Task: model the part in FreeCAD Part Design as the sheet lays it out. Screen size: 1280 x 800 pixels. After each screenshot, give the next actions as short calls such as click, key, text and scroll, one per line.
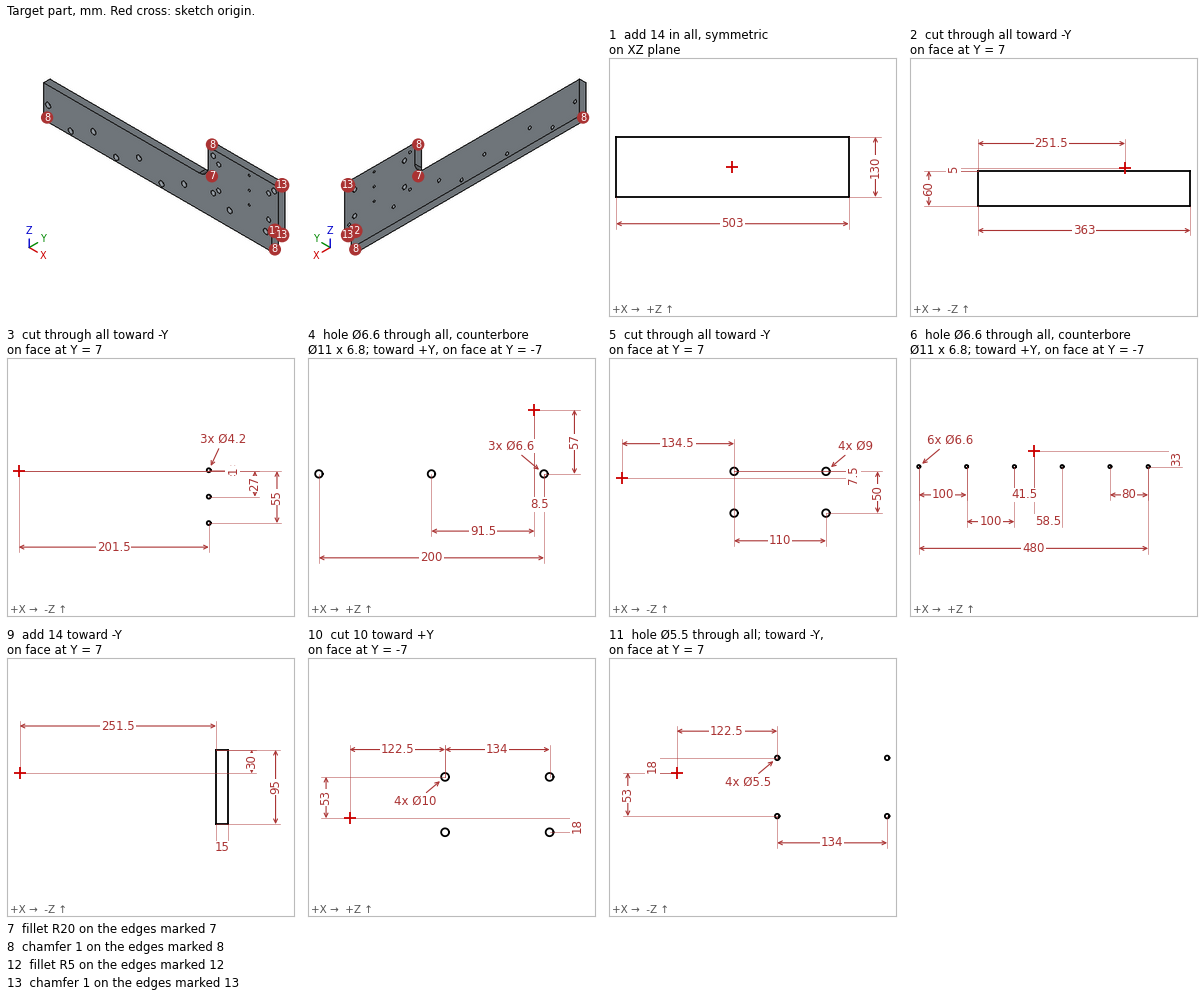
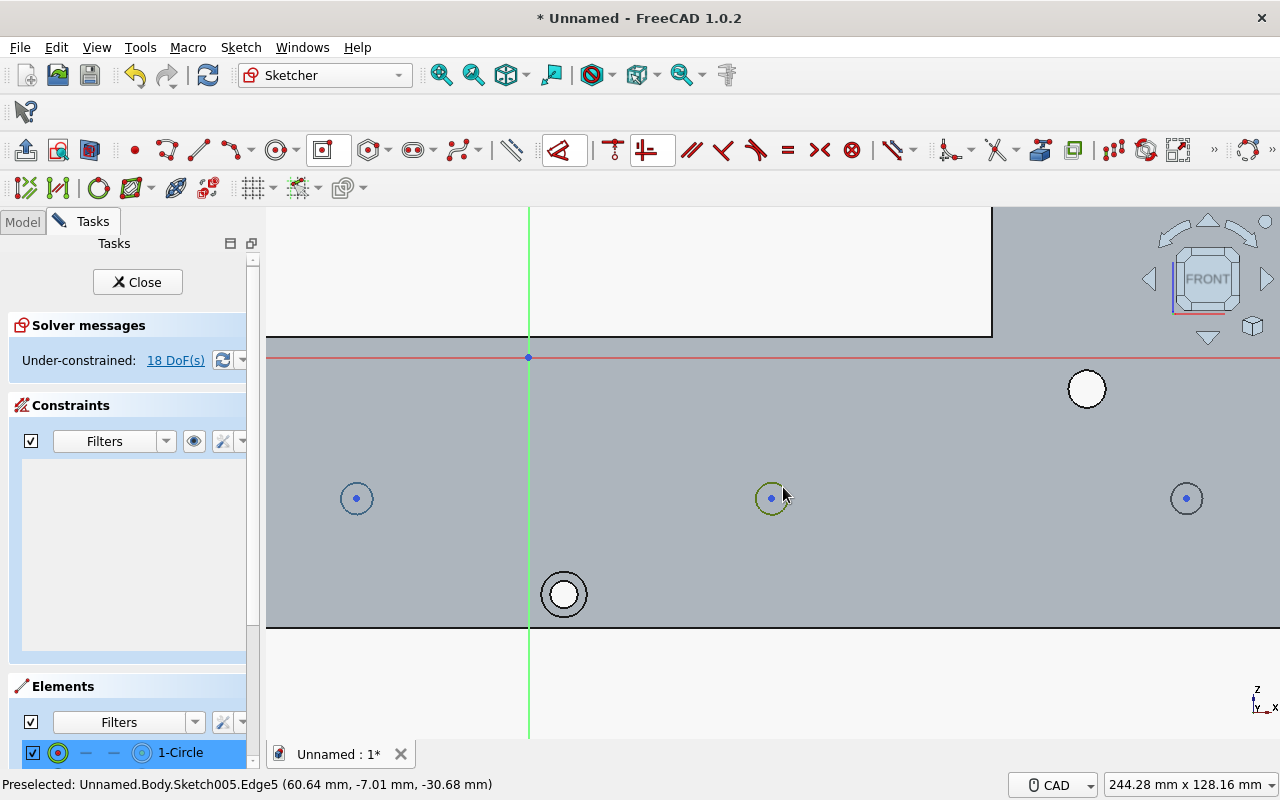
scroll(783, 490, down, 6)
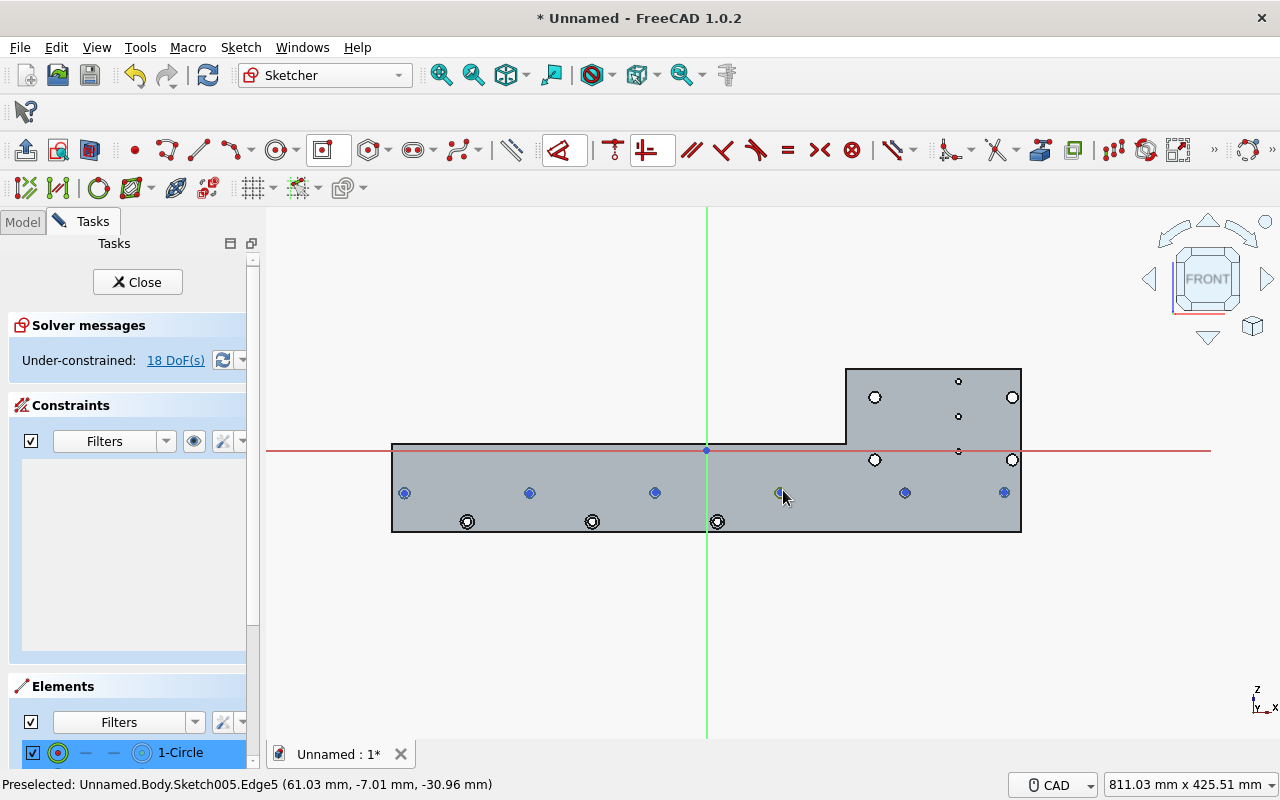
scroll(908, 490, up, 6)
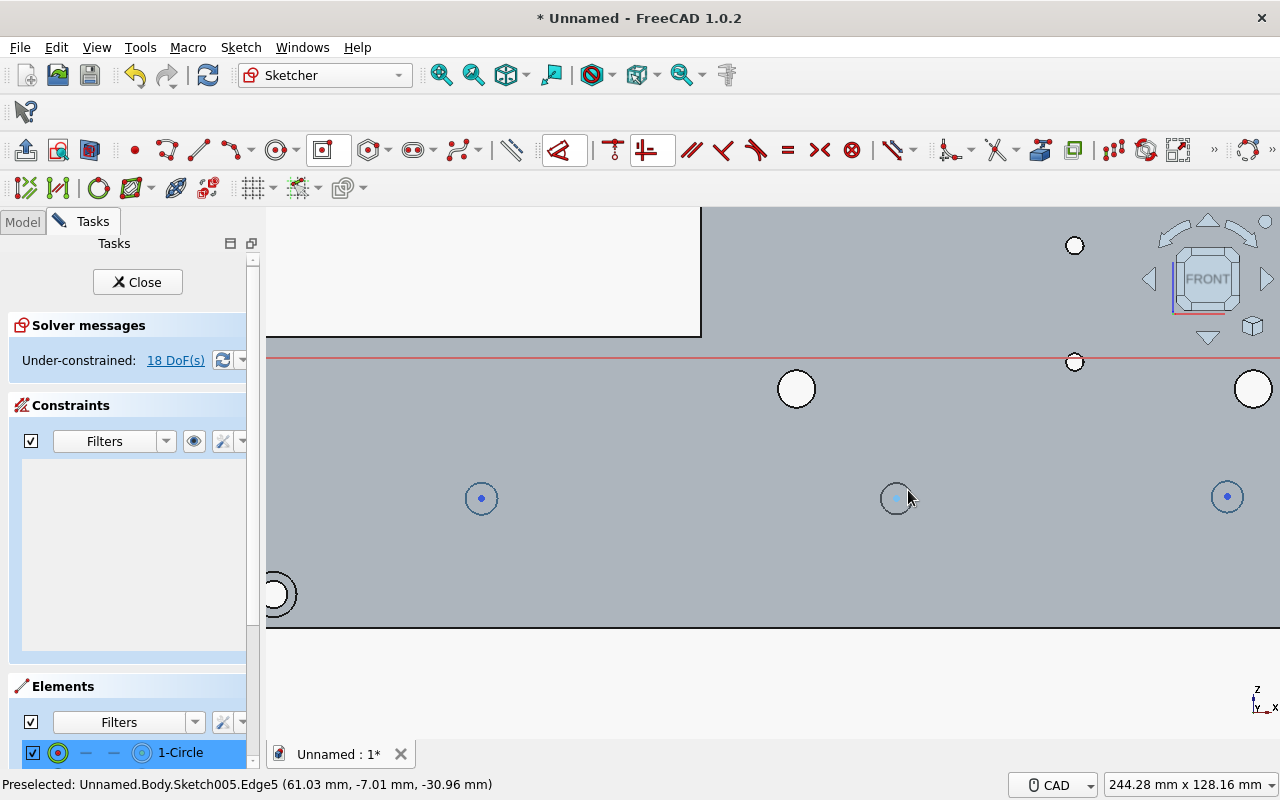
click(908, 488)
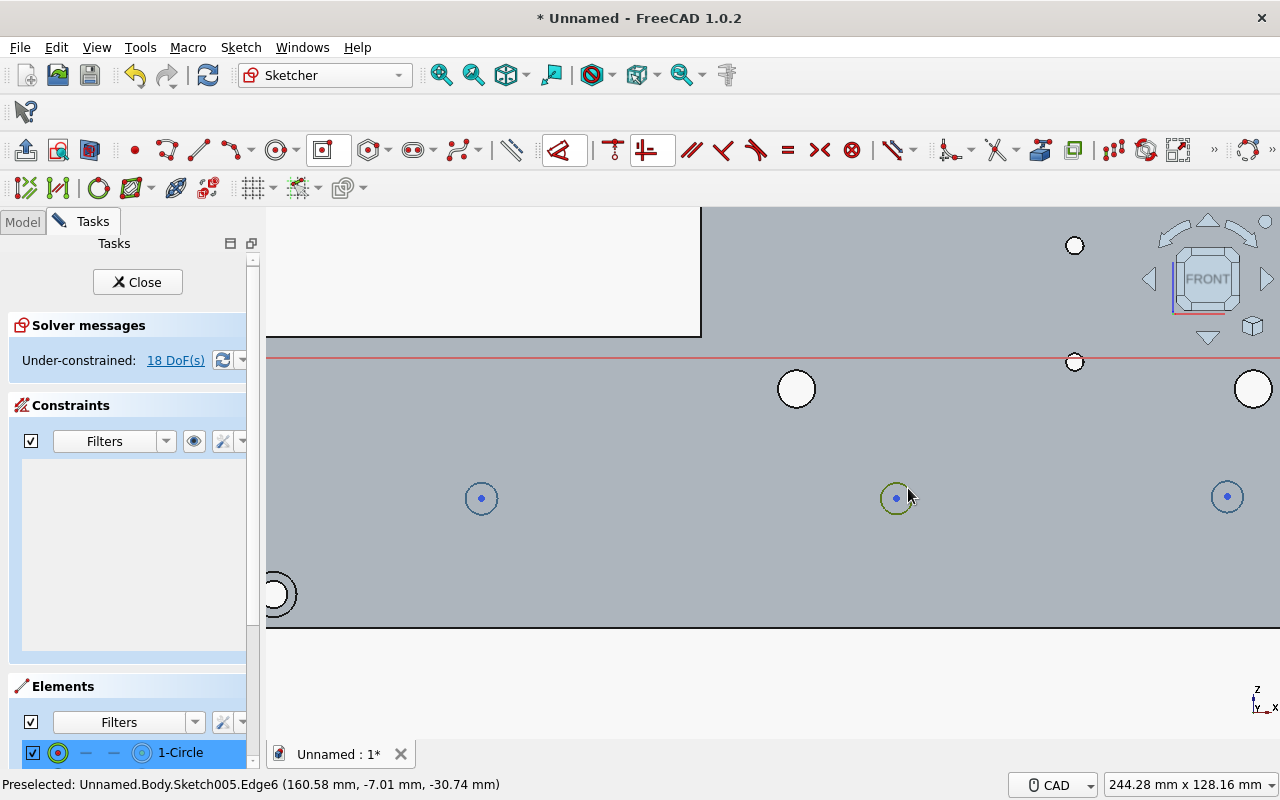
key(e)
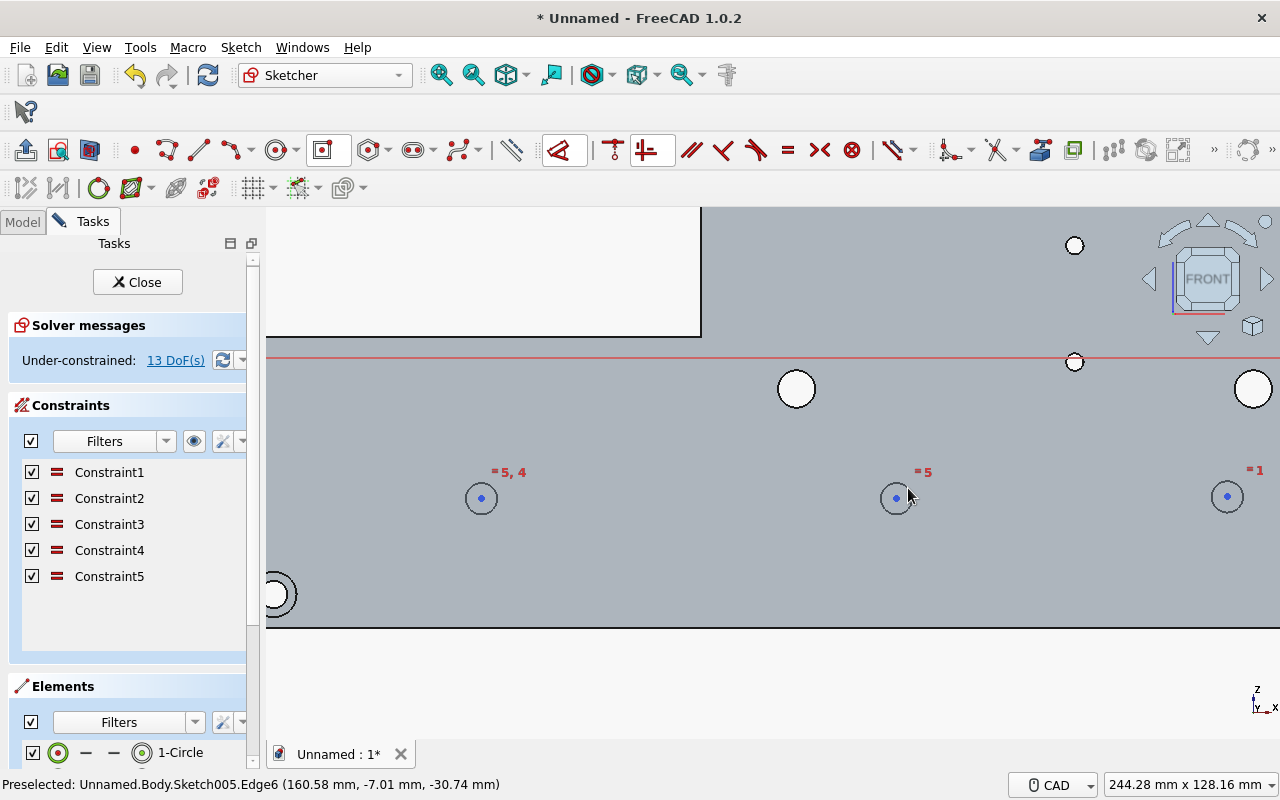
scroll(908, 490, down, 6)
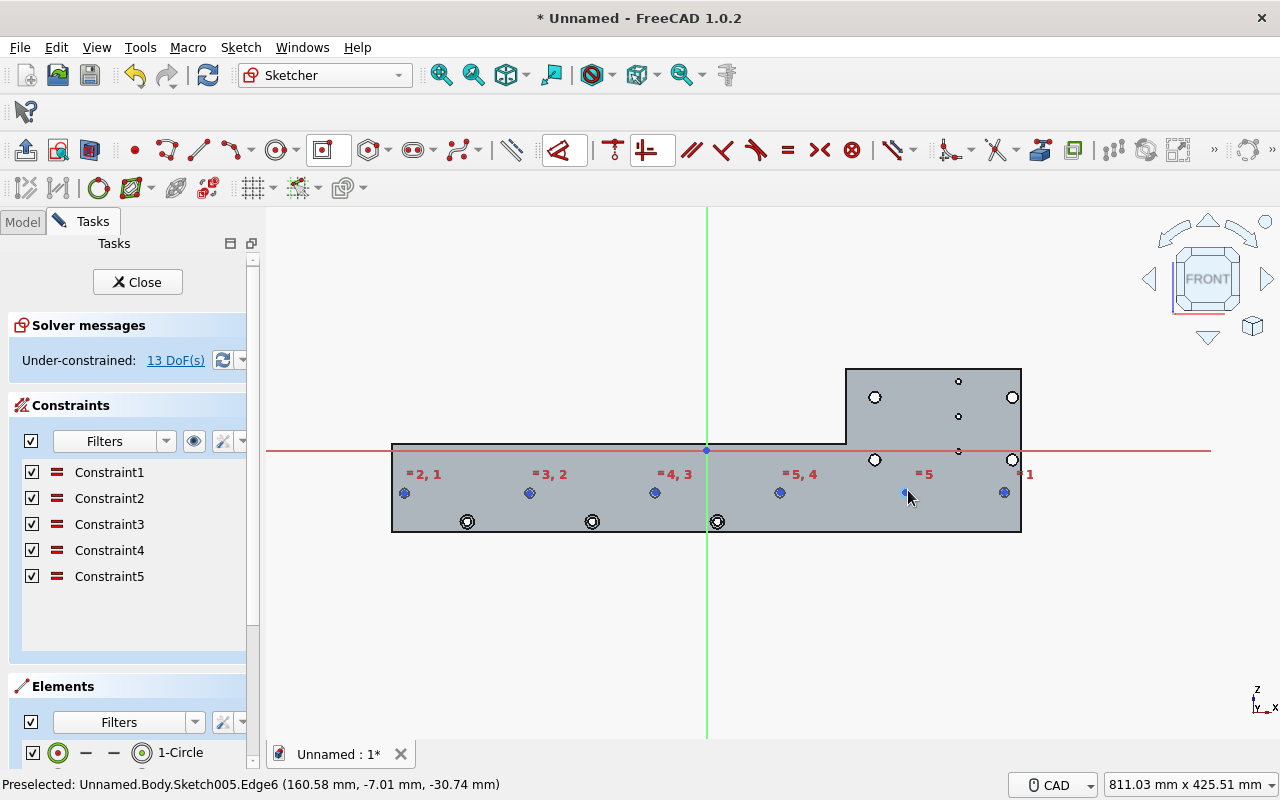
click(1005, 492)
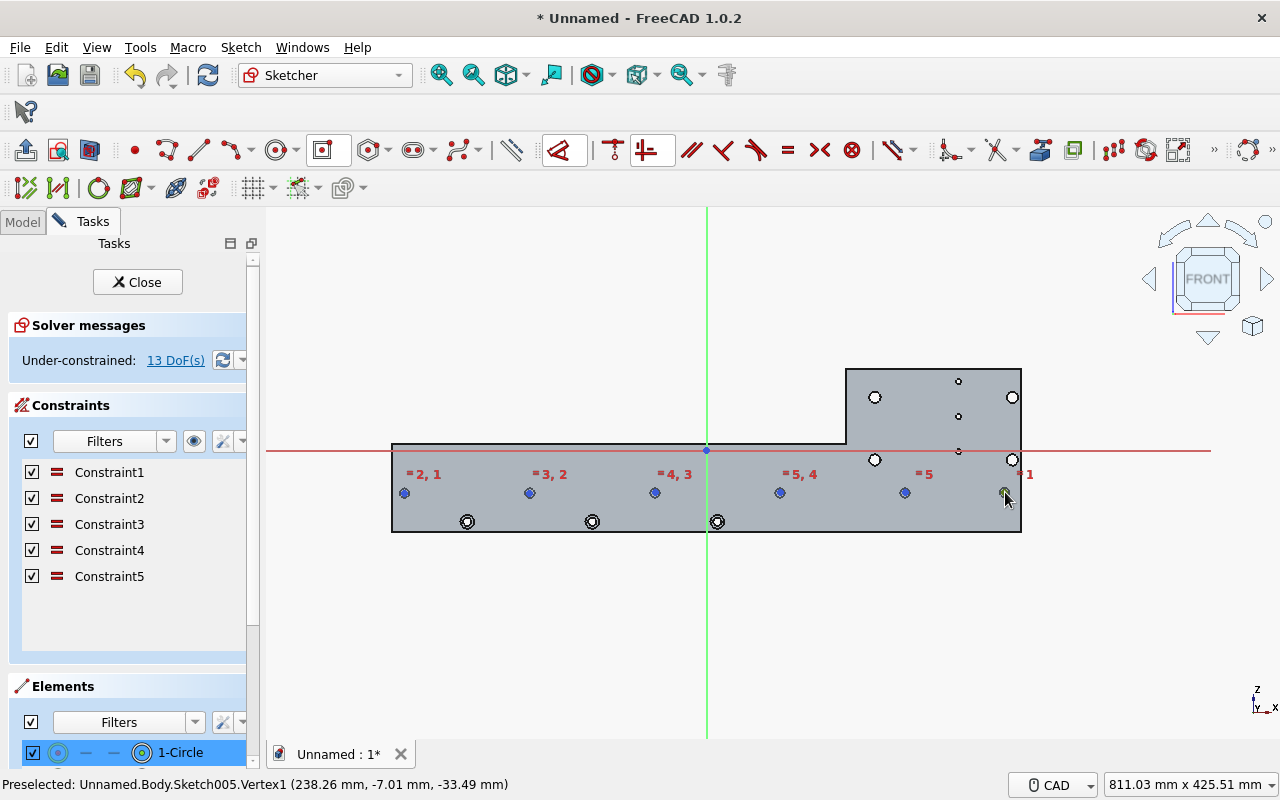
click(404, 493)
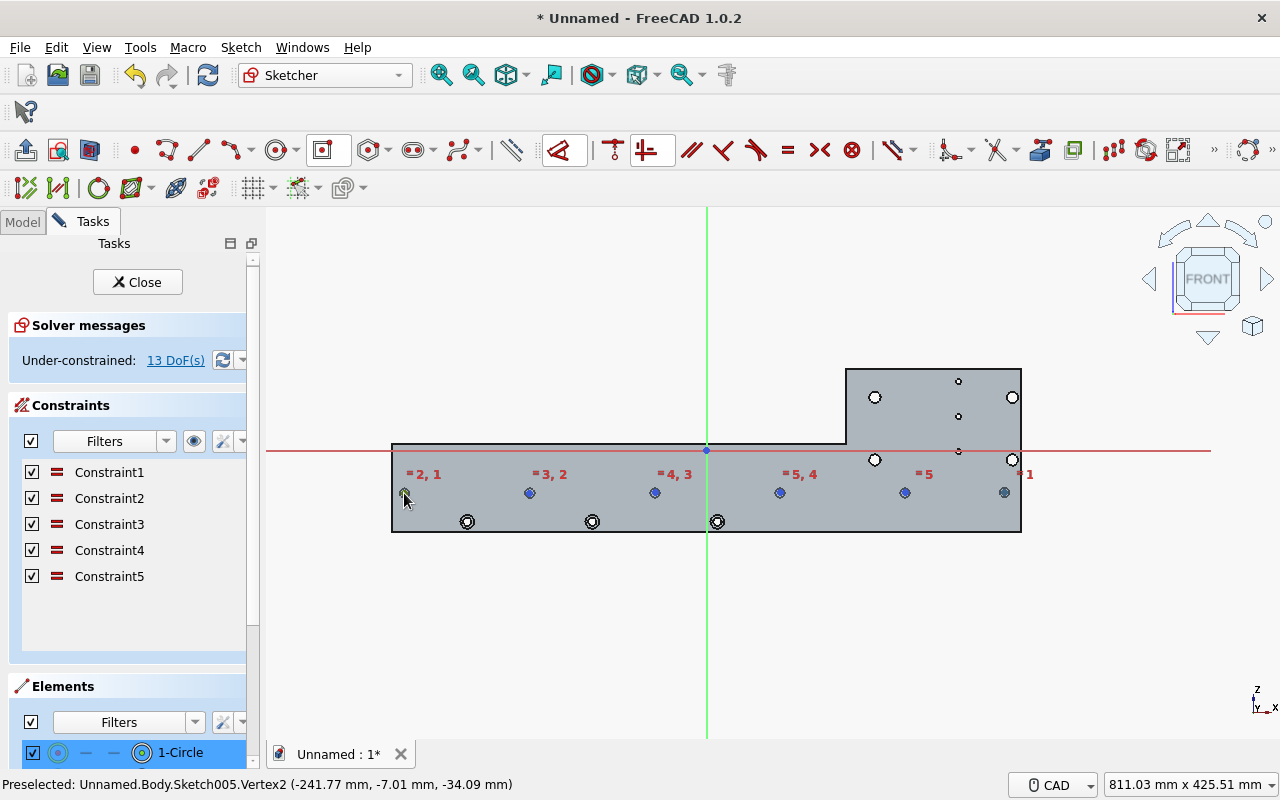
key(h)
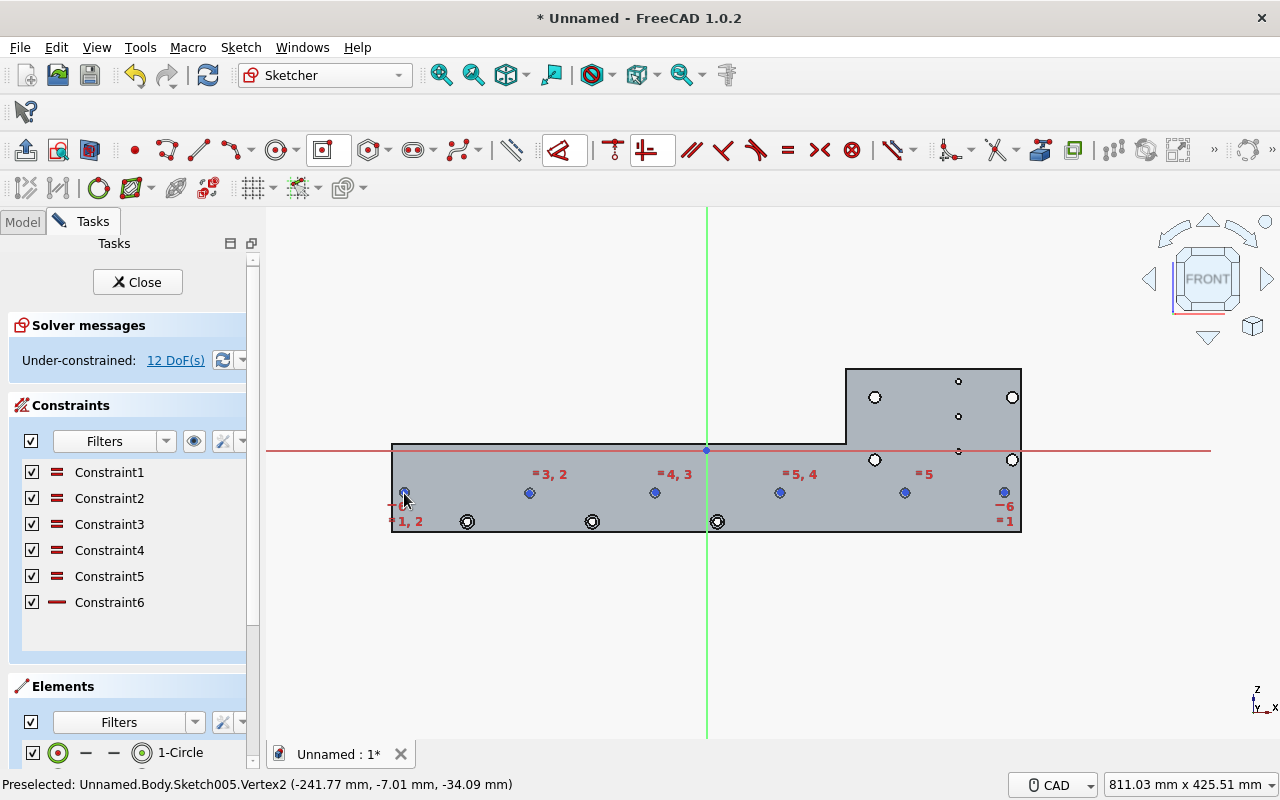
click(404, 492)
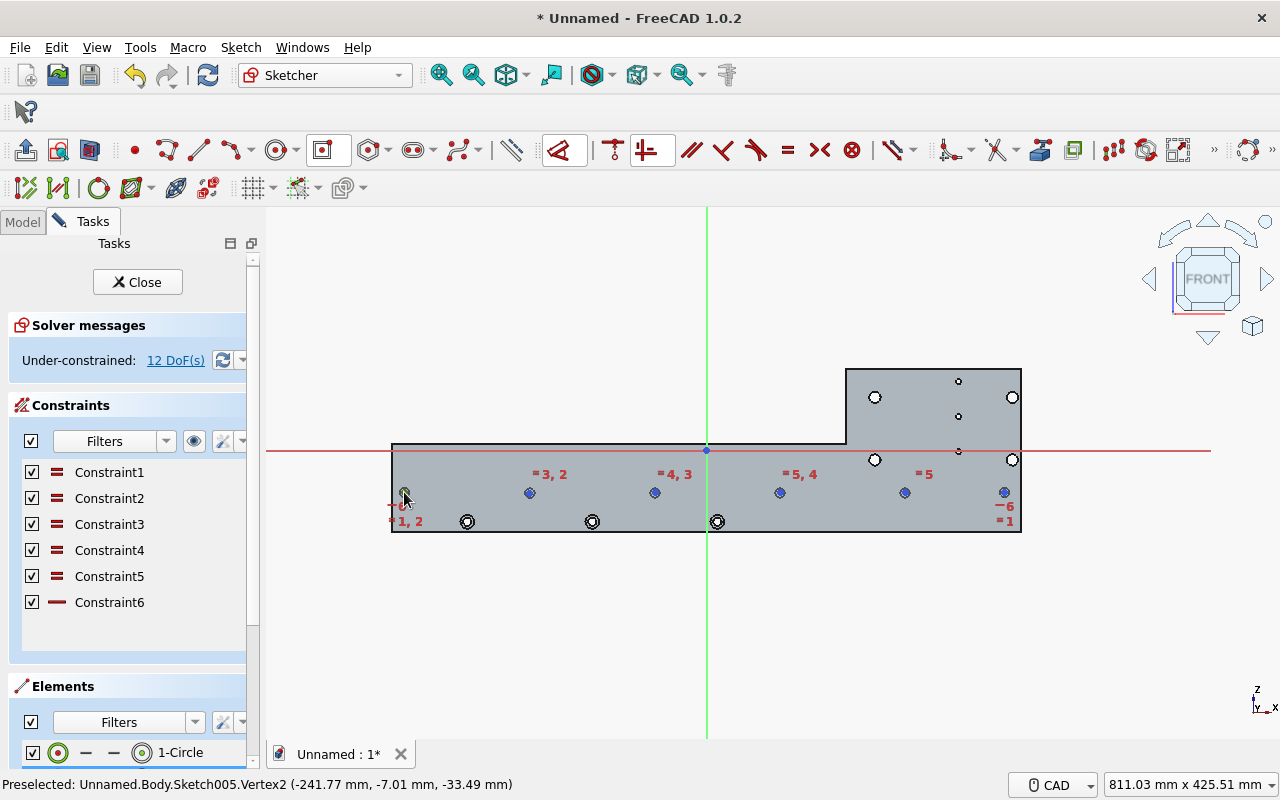
click(530, 493)